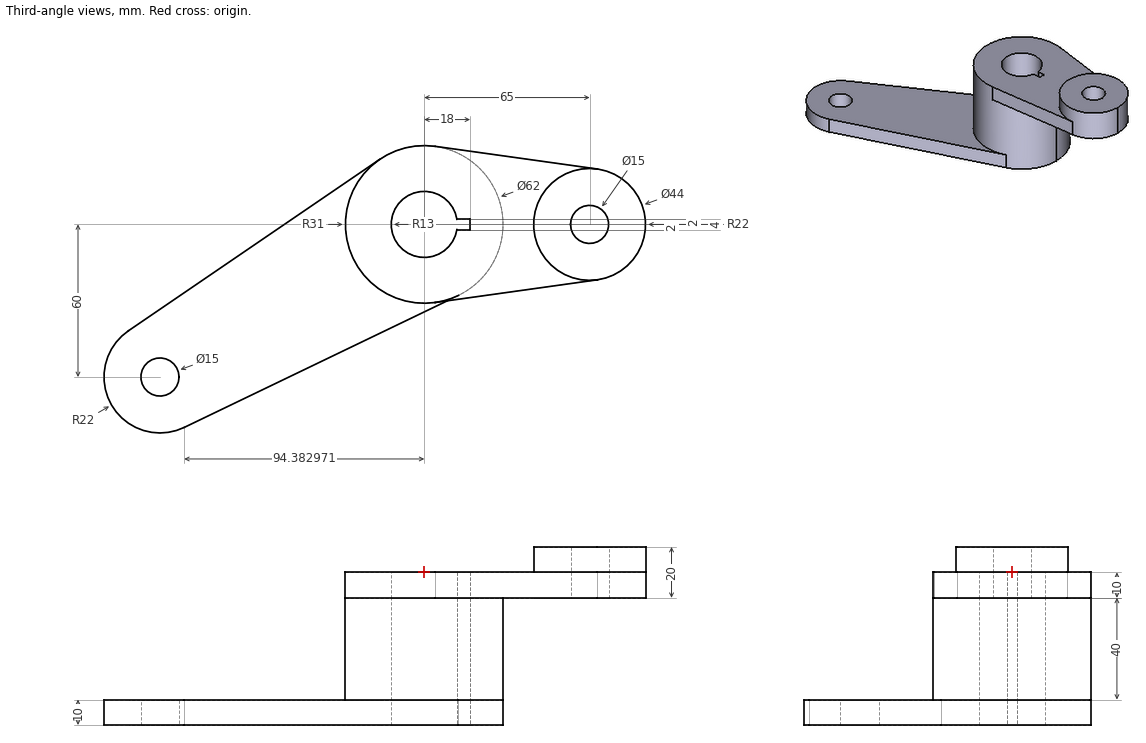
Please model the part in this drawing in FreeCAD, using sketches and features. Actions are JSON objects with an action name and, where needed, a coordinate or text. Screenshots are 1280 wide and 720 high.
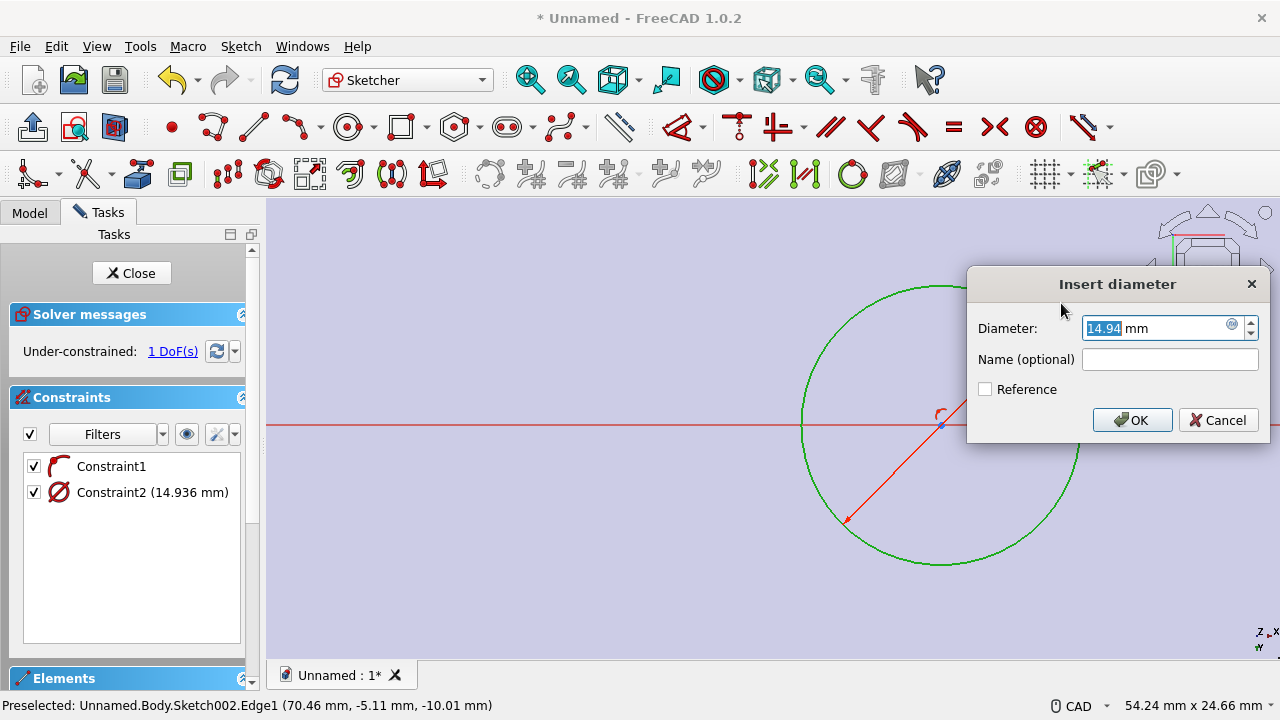
{"action": "type", "text": "15"}
{"action": "key", "text": "Return"}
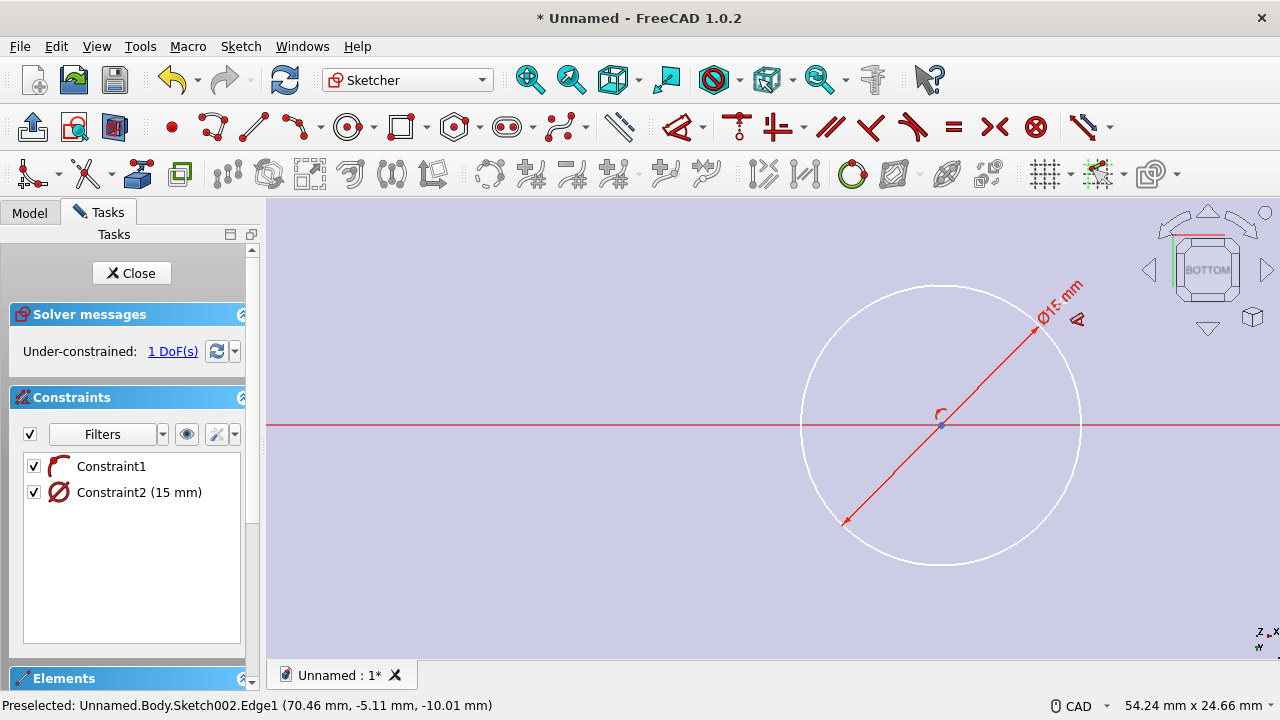
{"action": "left_click", "coordinate": [941, 425]}
{"action": "left_click", "coordinate": [618, 459]}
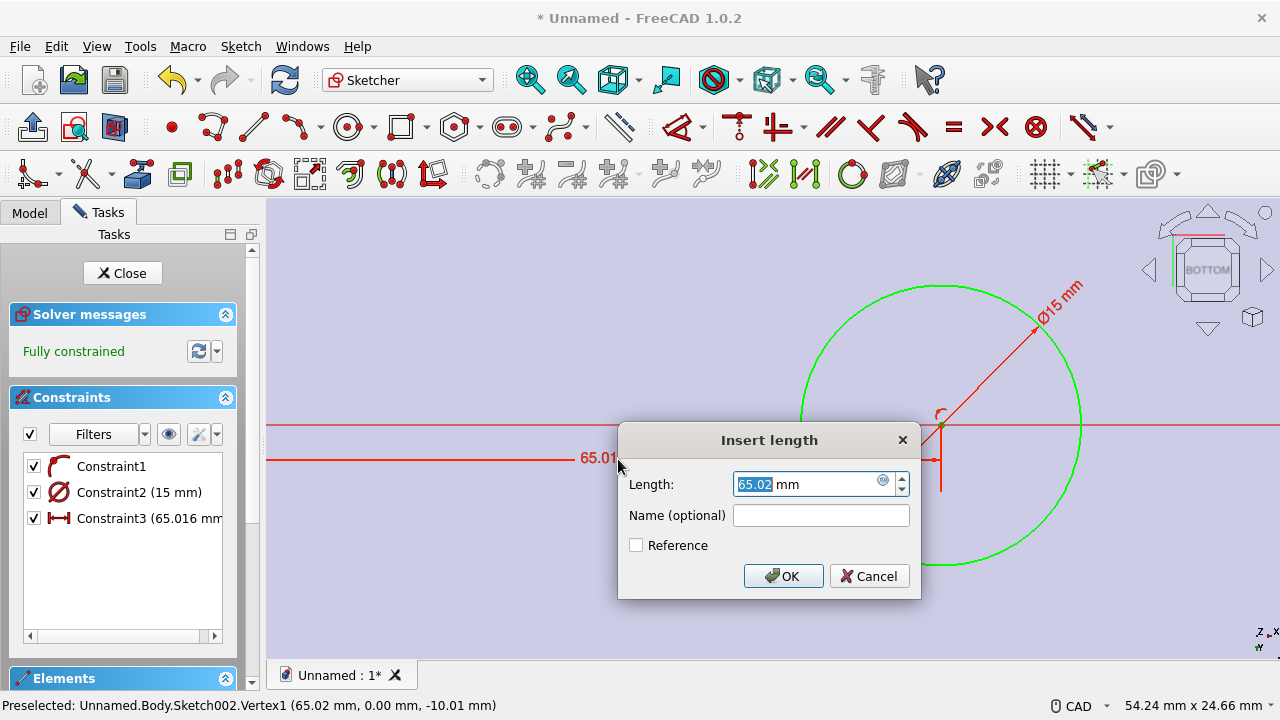
{"action": "type", "text": "65"}
{"action": "key", "text": "Return"}
{"action": "key", "text": "Escape"}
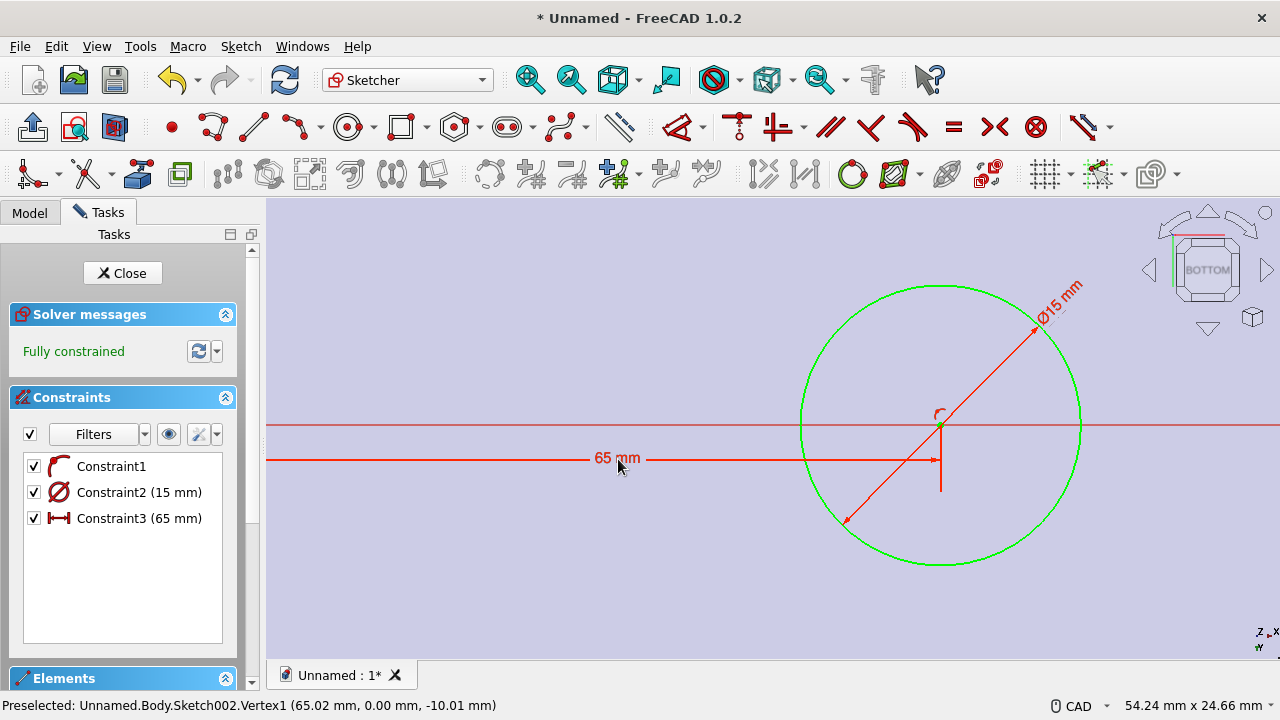
{"action": "left_click", "coordinate": [123, 273]}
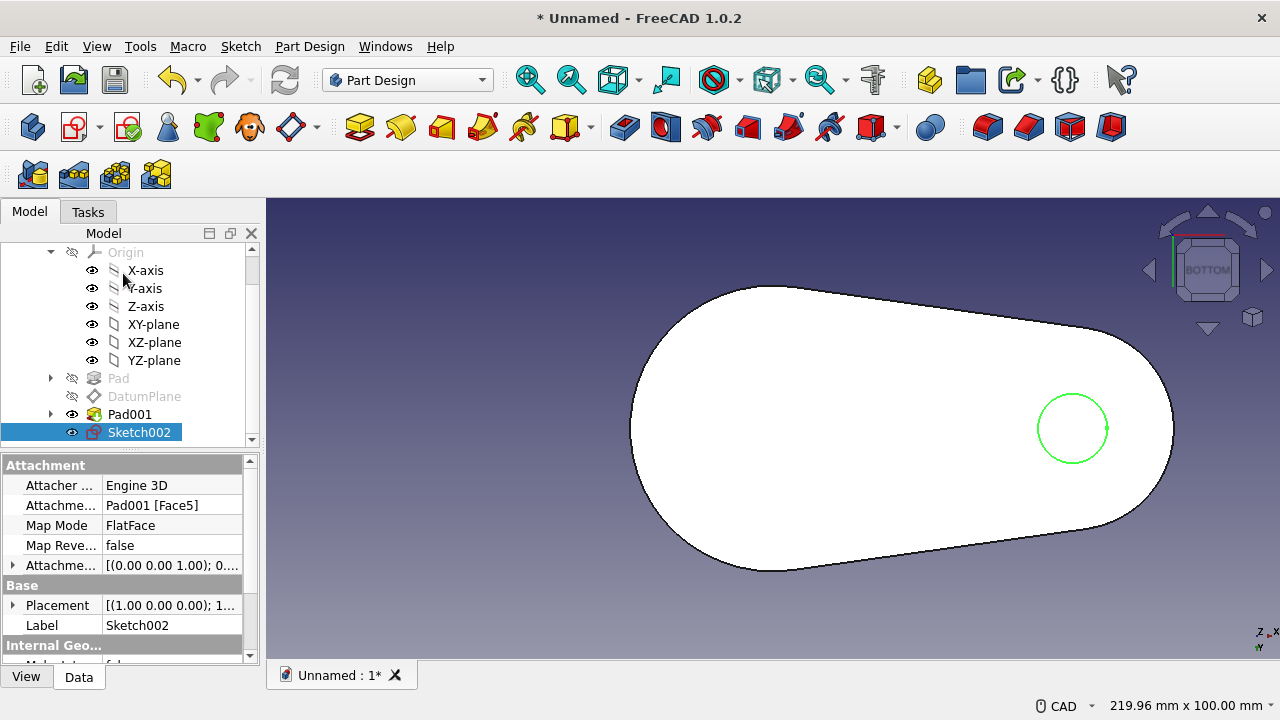
{"action": "left_click", "coordinate": [625, 128]}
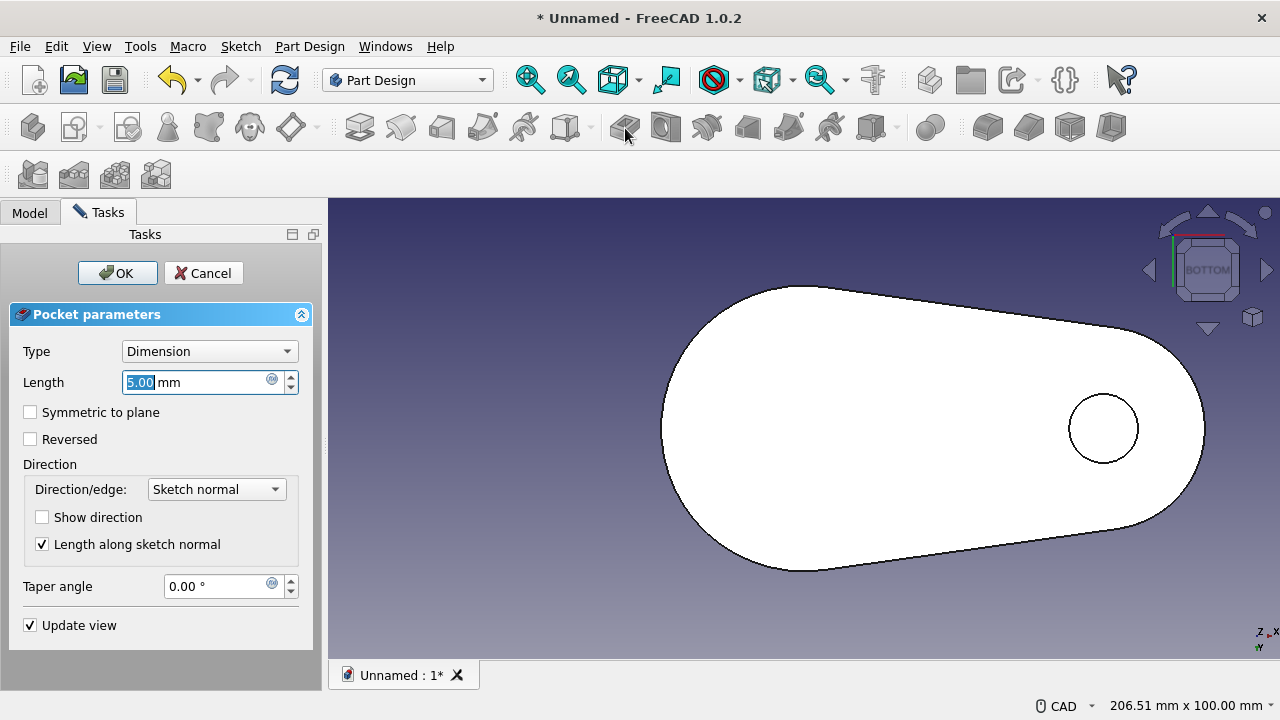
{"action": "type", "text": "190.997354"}
{"action": "key", "text": "Tab"}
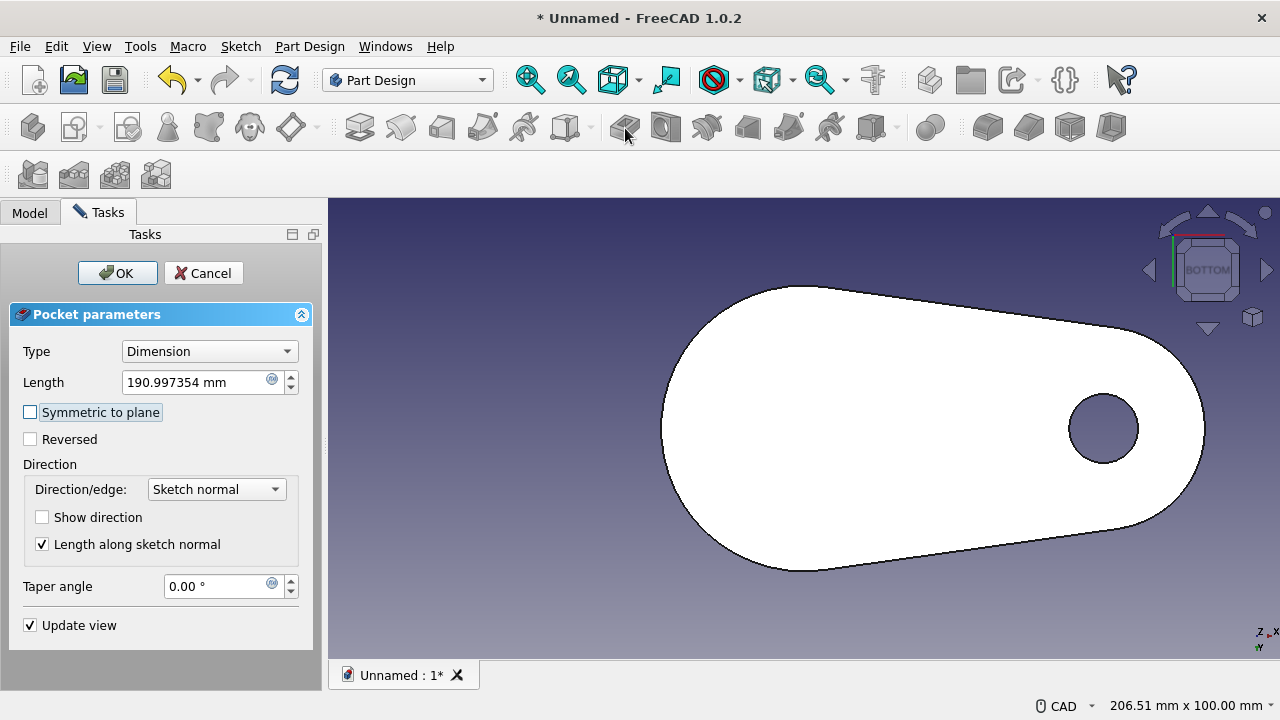
{"action": "left_click", "coordinate": [31, 412]}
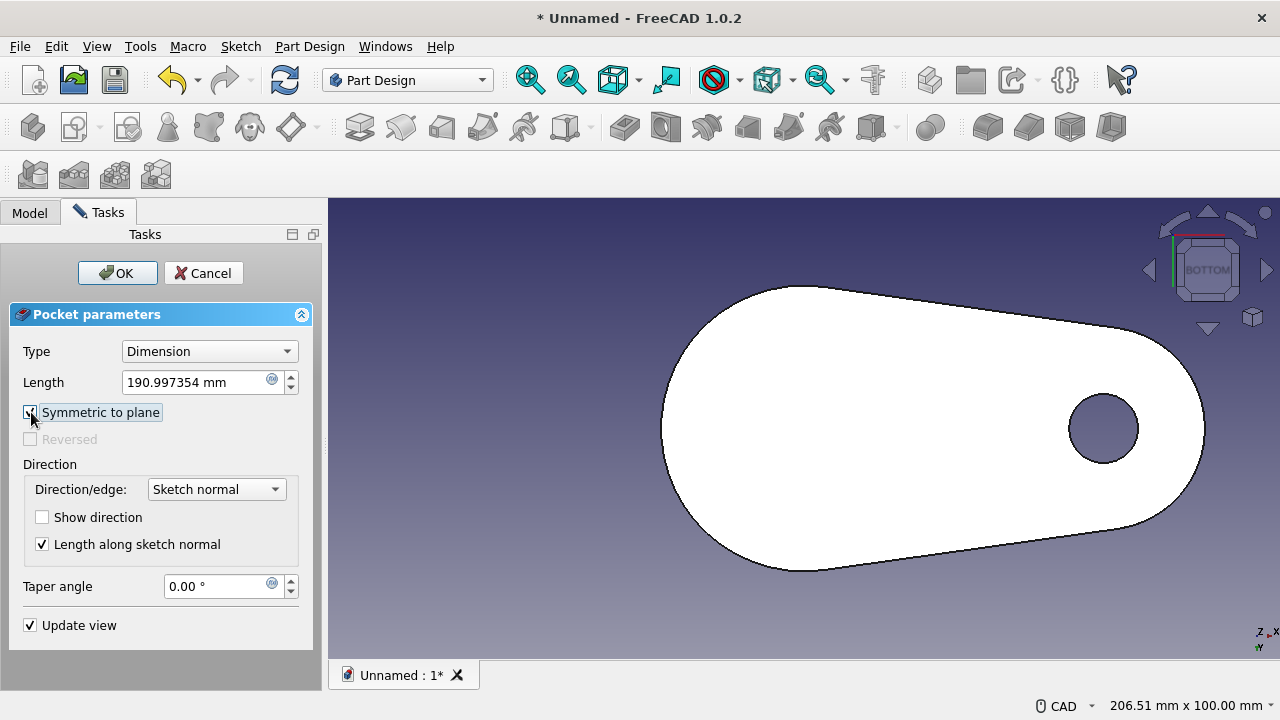
{"action": "left_click", "coordinate": [118, 273]}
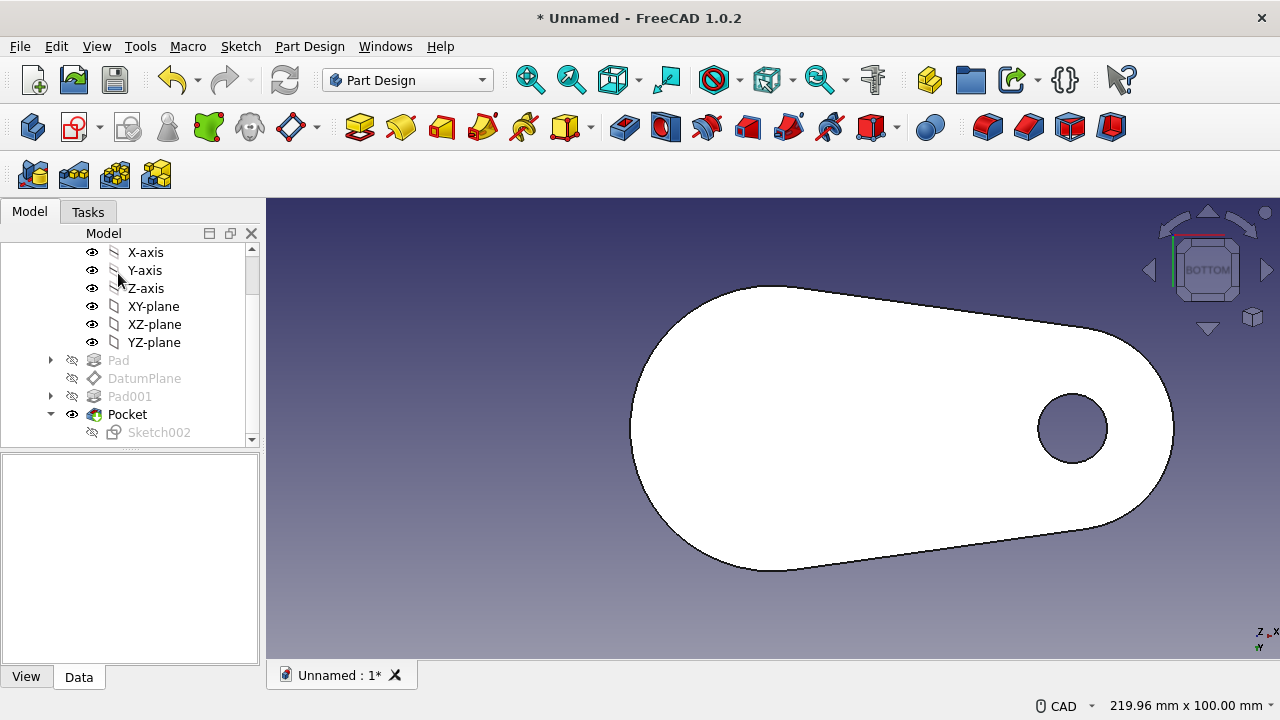
{"action": "left_click", "coordinate": [824, 428]}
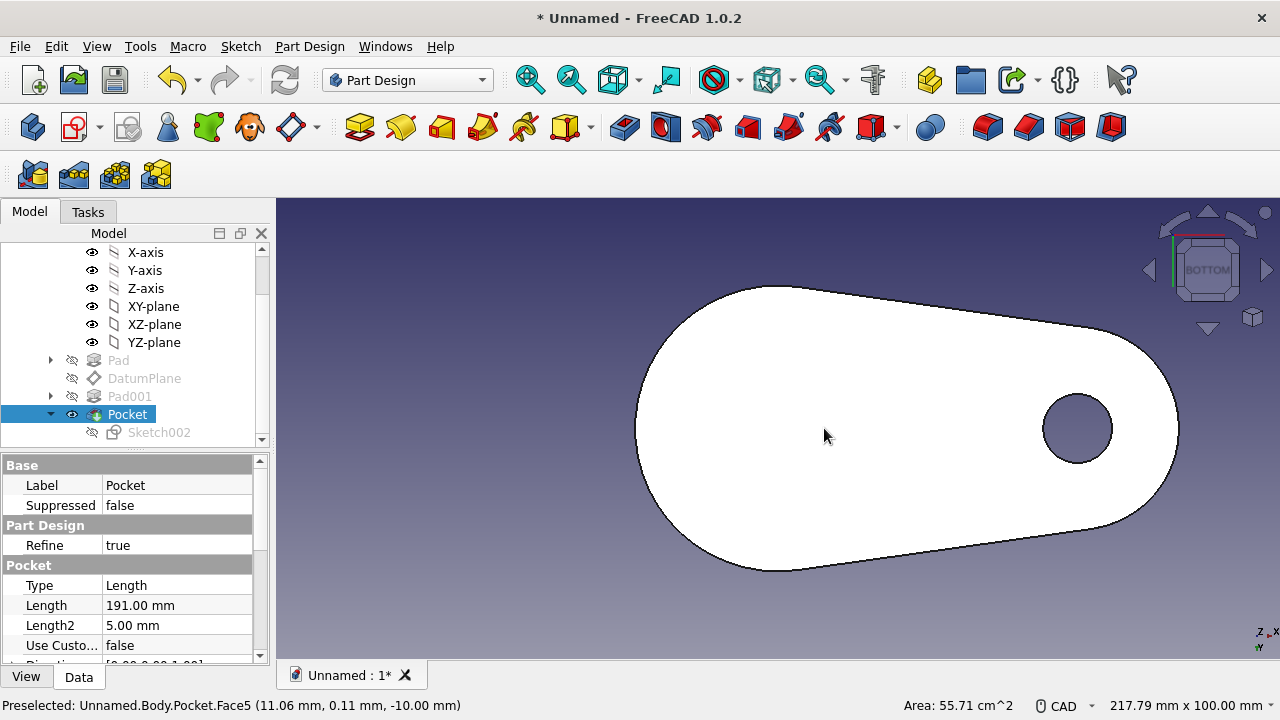
{"action": "left_click", "coordinate": [74, 128]}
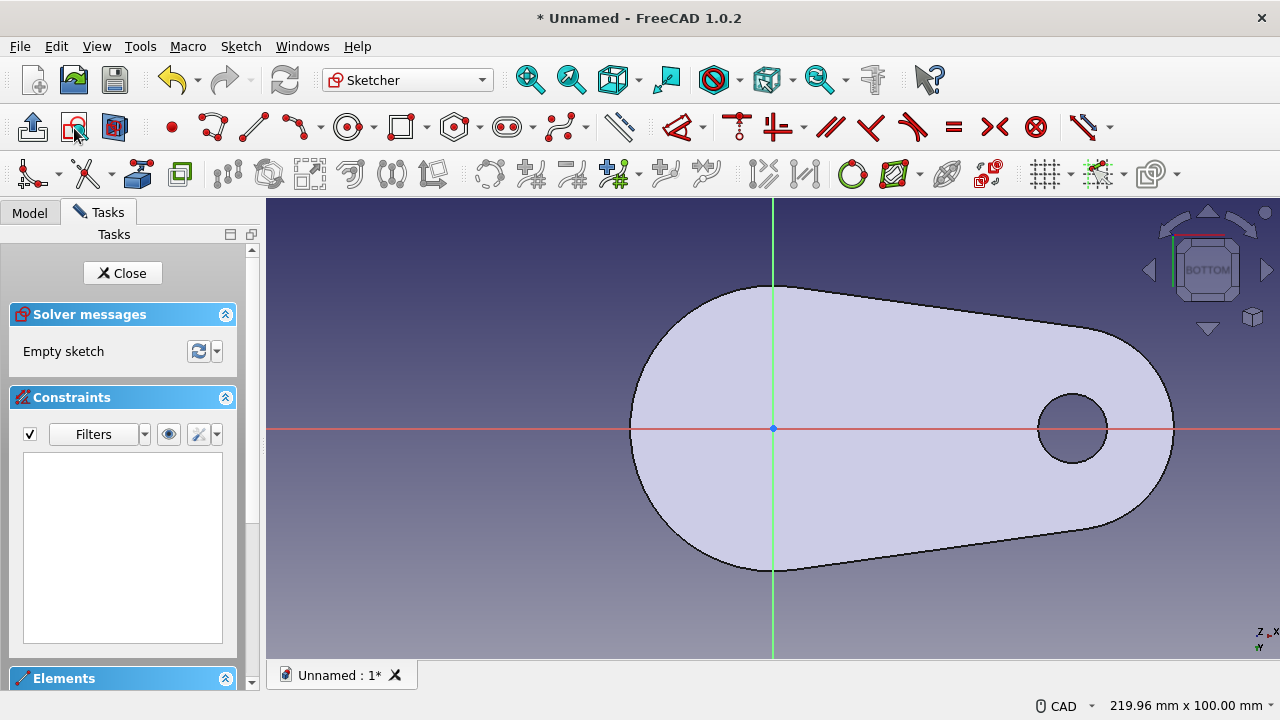
{"action": "key", "text": "g m"}